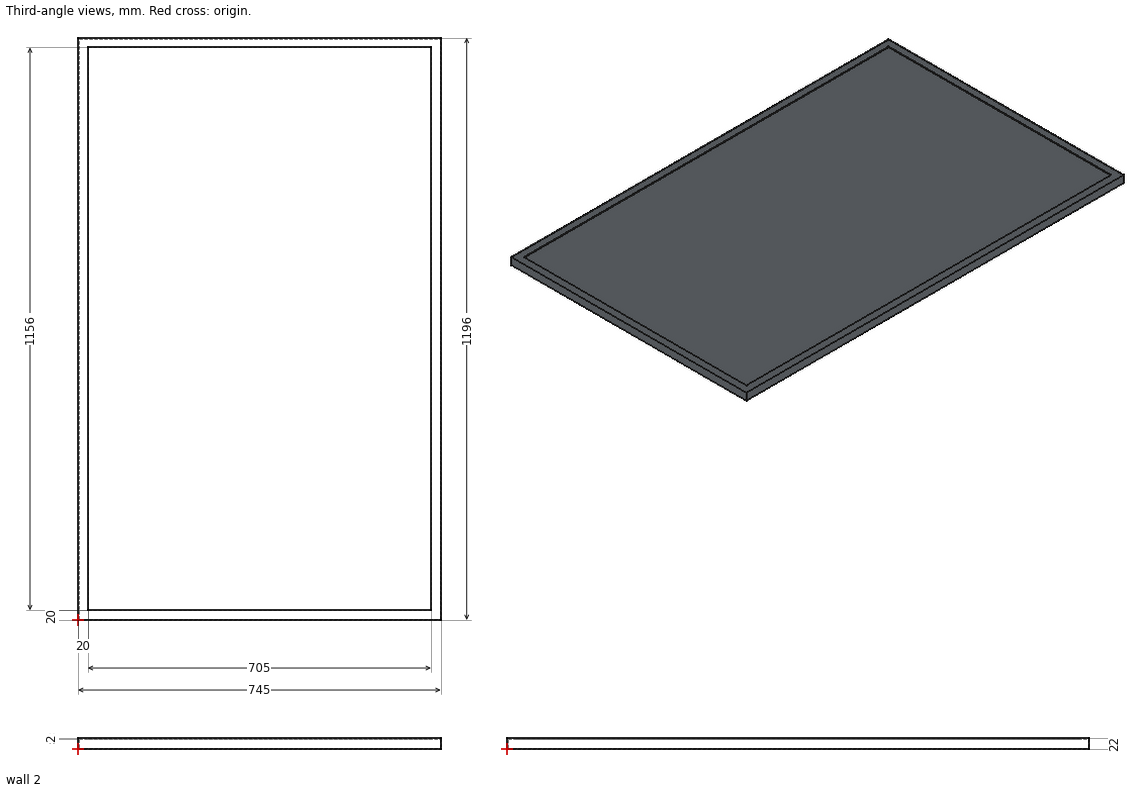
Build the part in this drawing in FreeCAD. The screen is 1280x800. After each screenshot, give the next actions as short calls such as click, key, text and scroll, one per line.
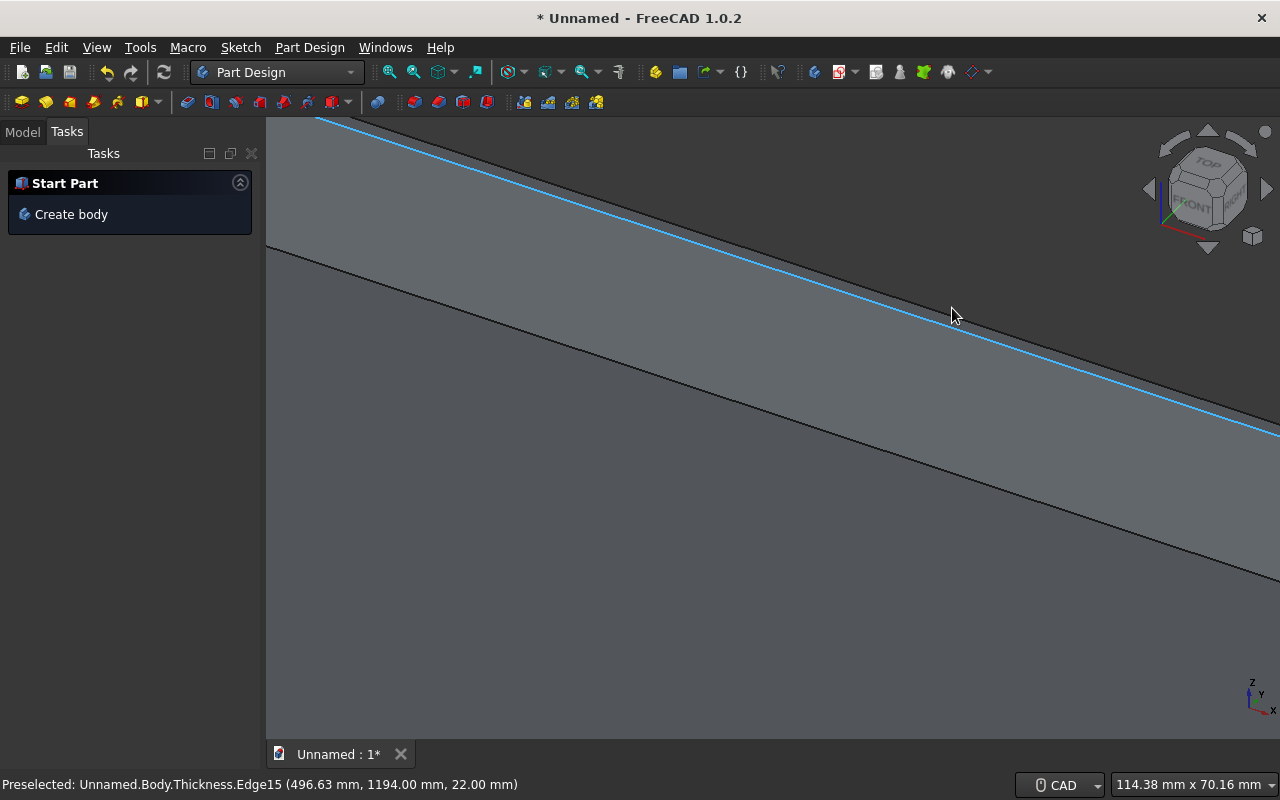
scroll(942, 320, up, 4)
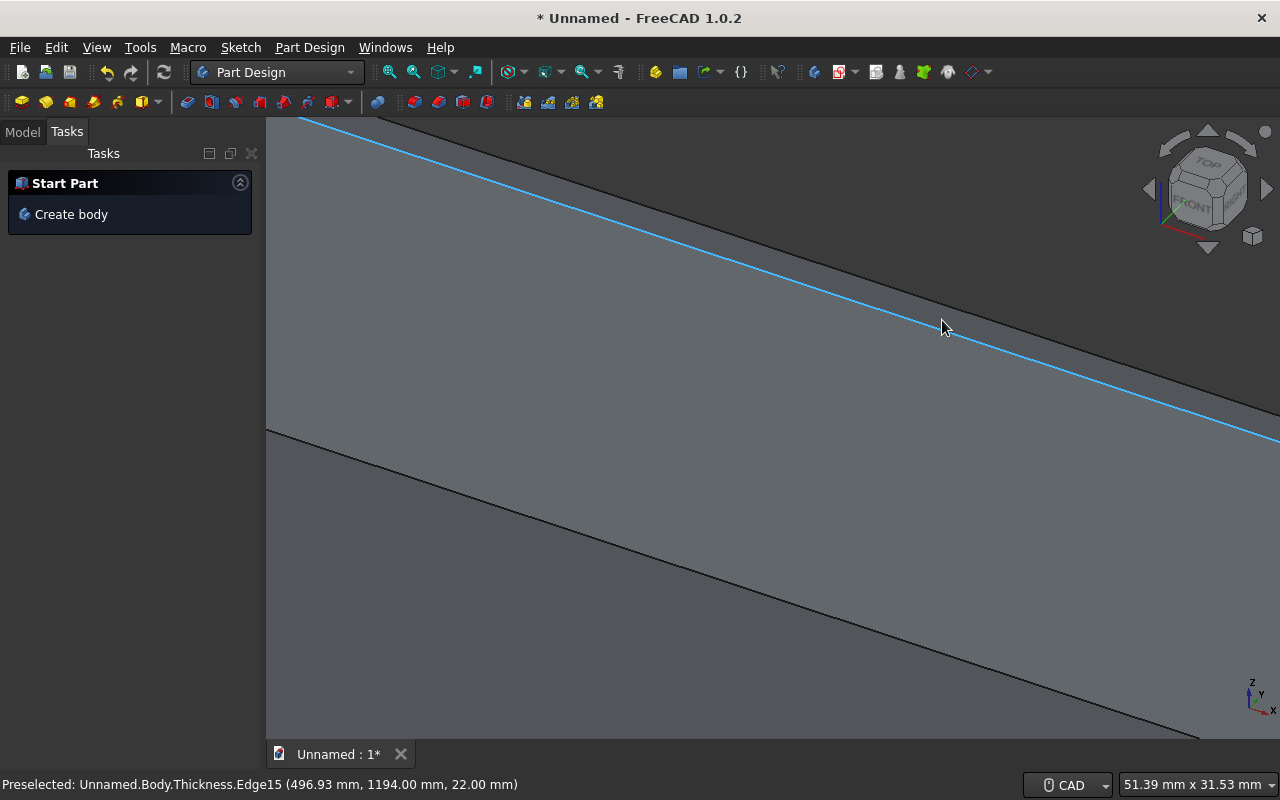
click(390, 72)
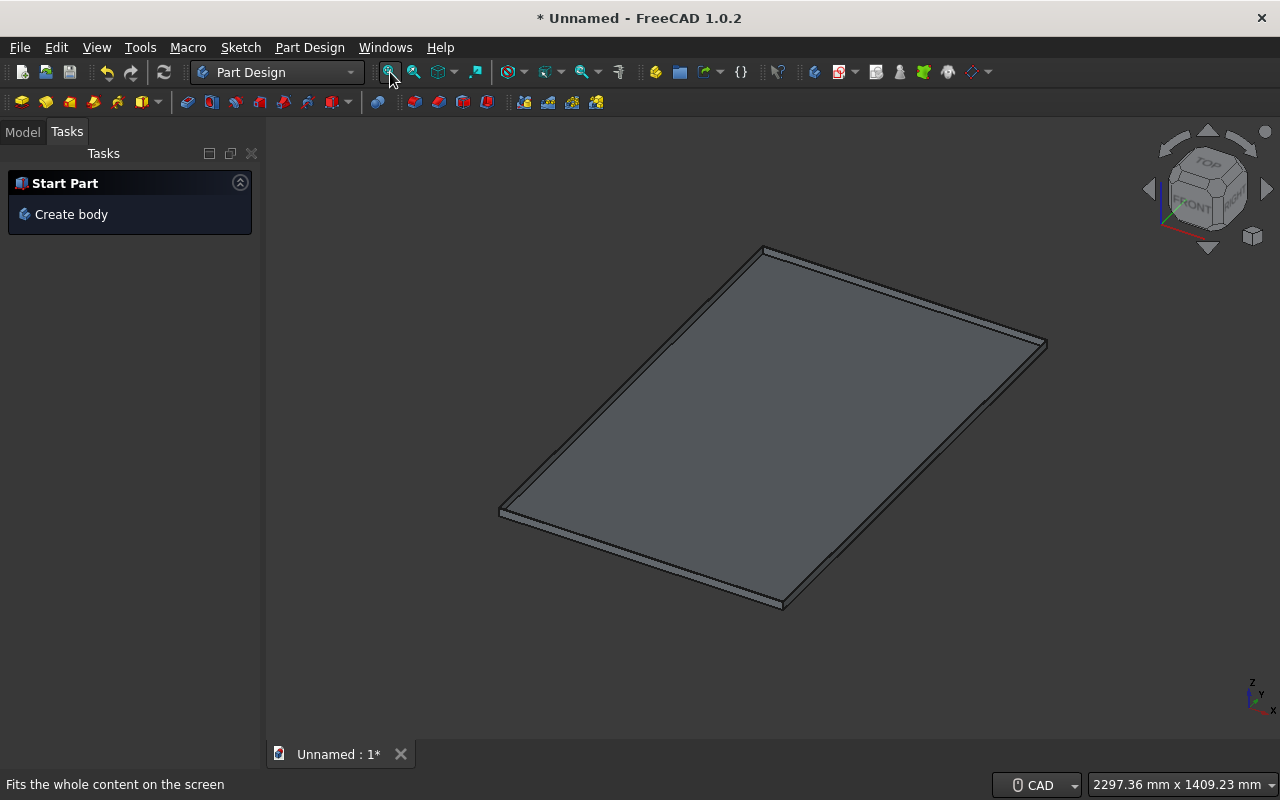
key(0)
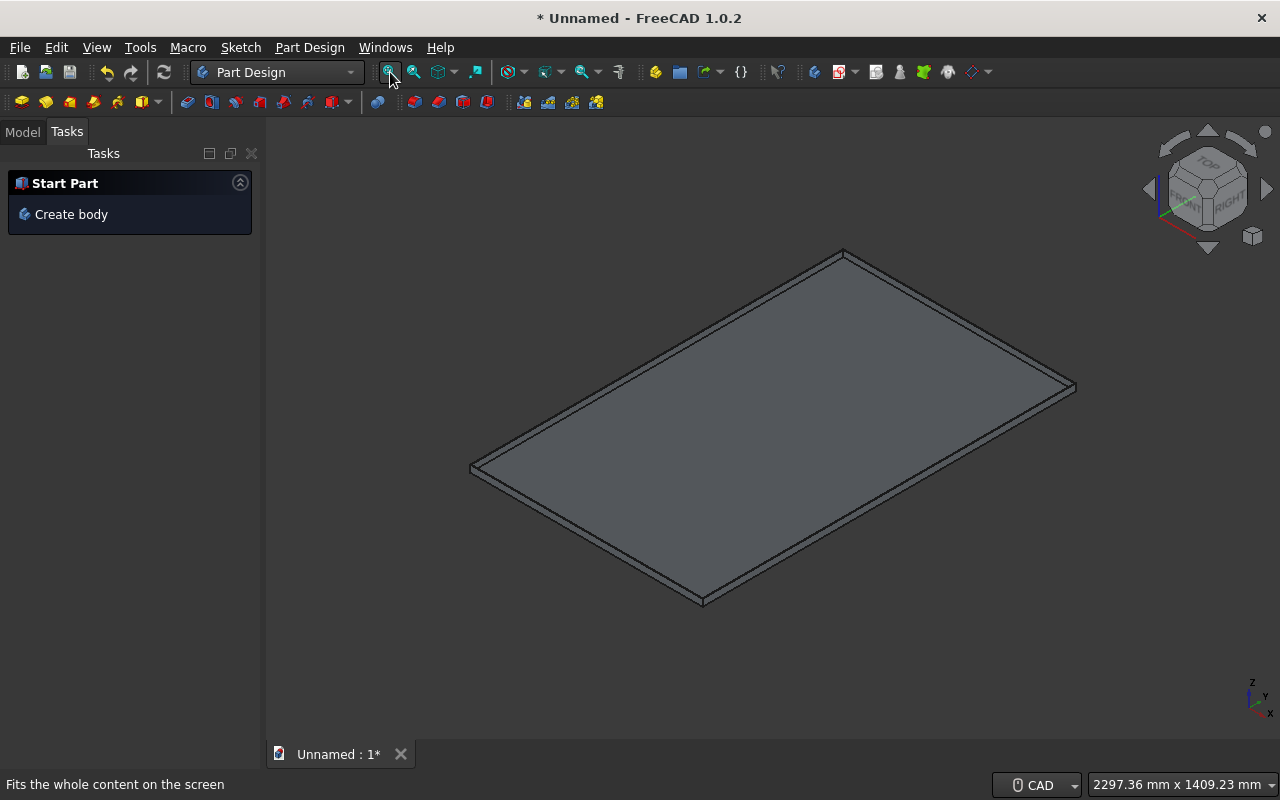
scroll(998, 338, up, 15)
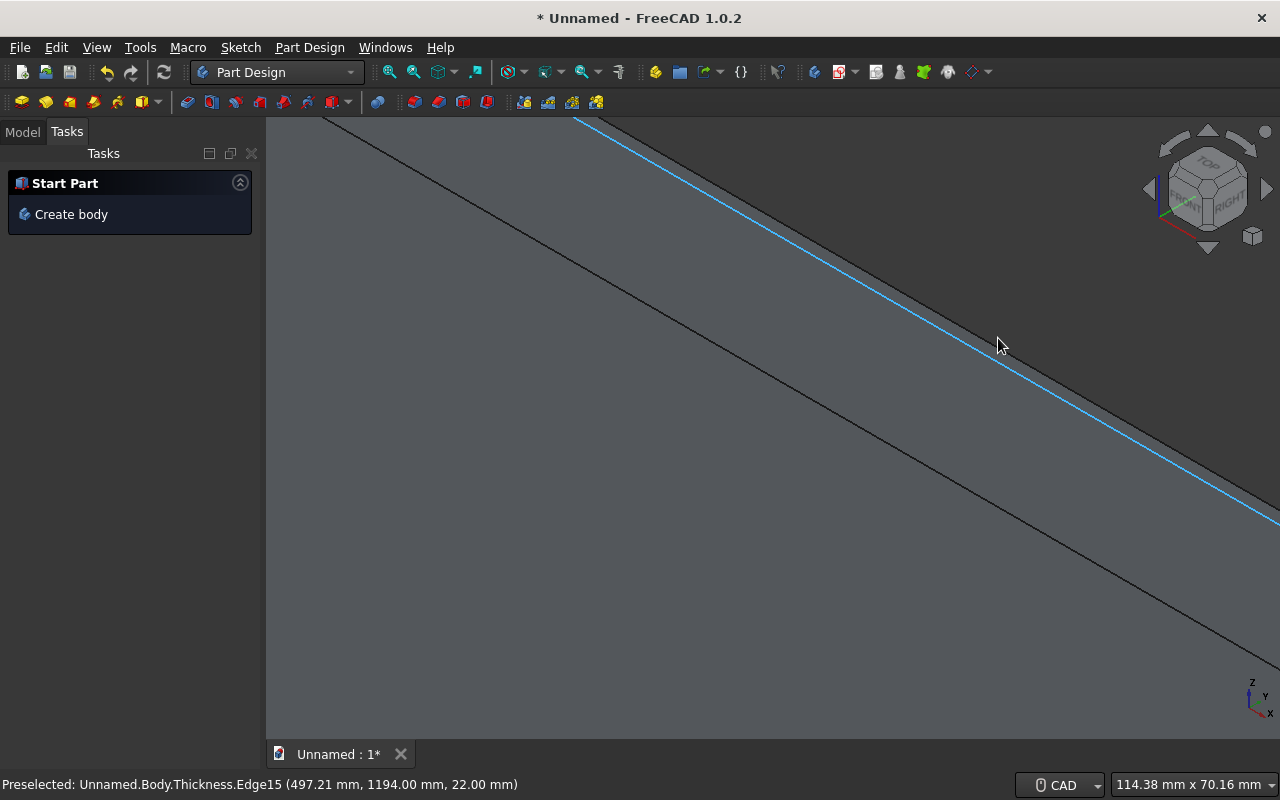
scroll(984, 348, up, 4)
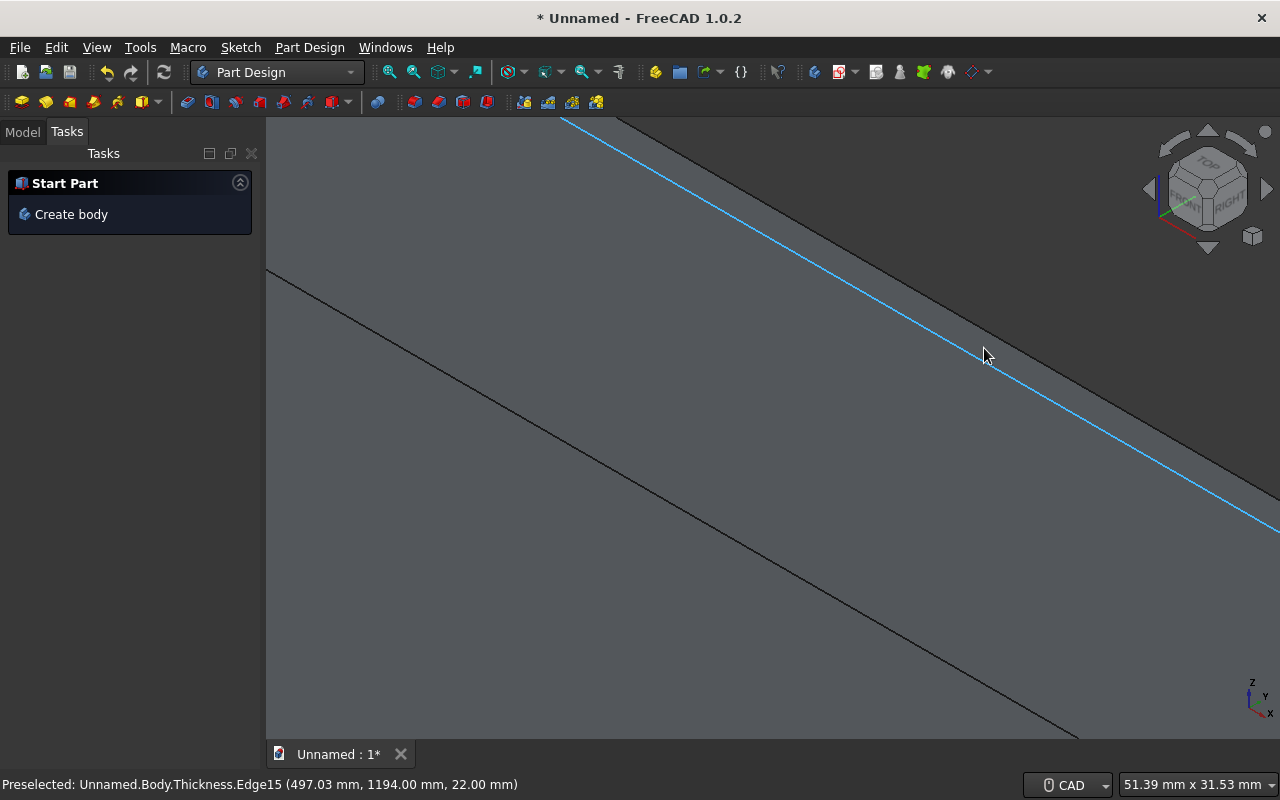
click(982, 349)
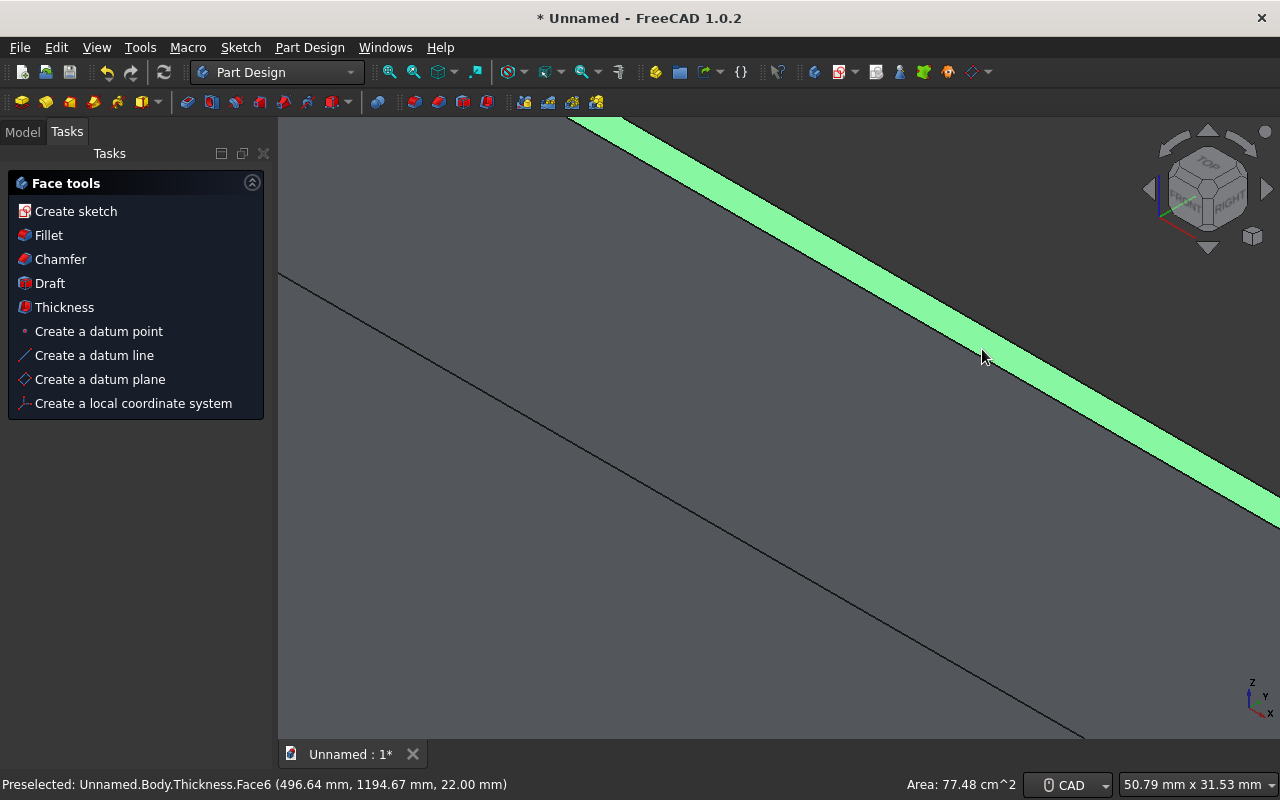
click(840, 72)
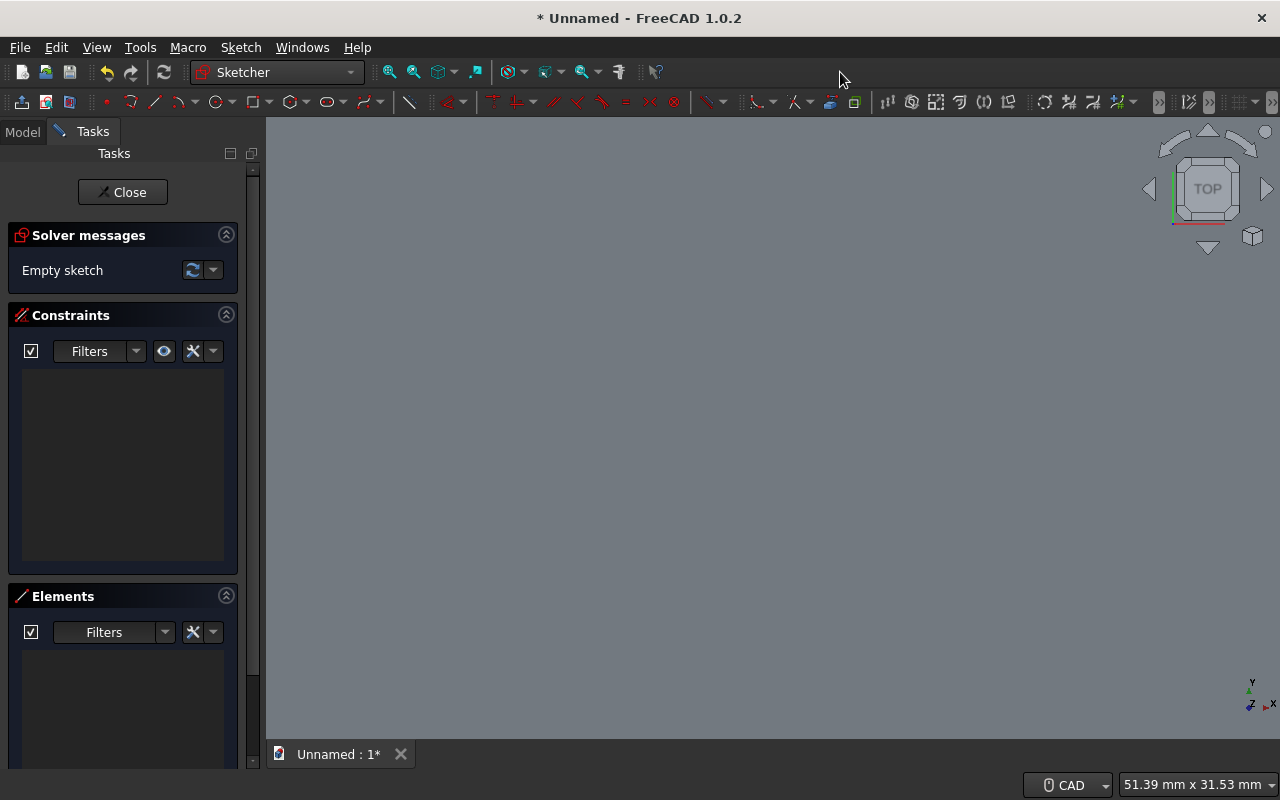
scroll(704, 428, down, 15)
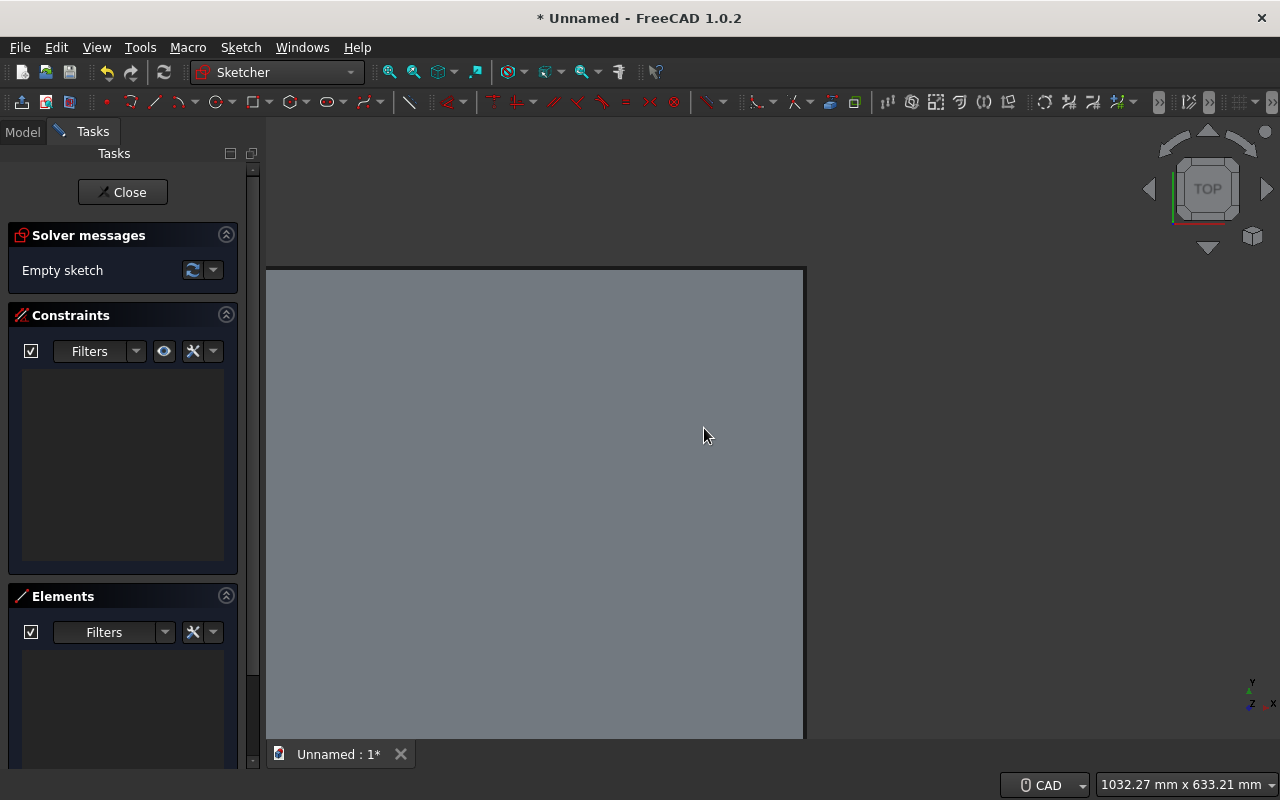
scroll(858, 180, down, 5)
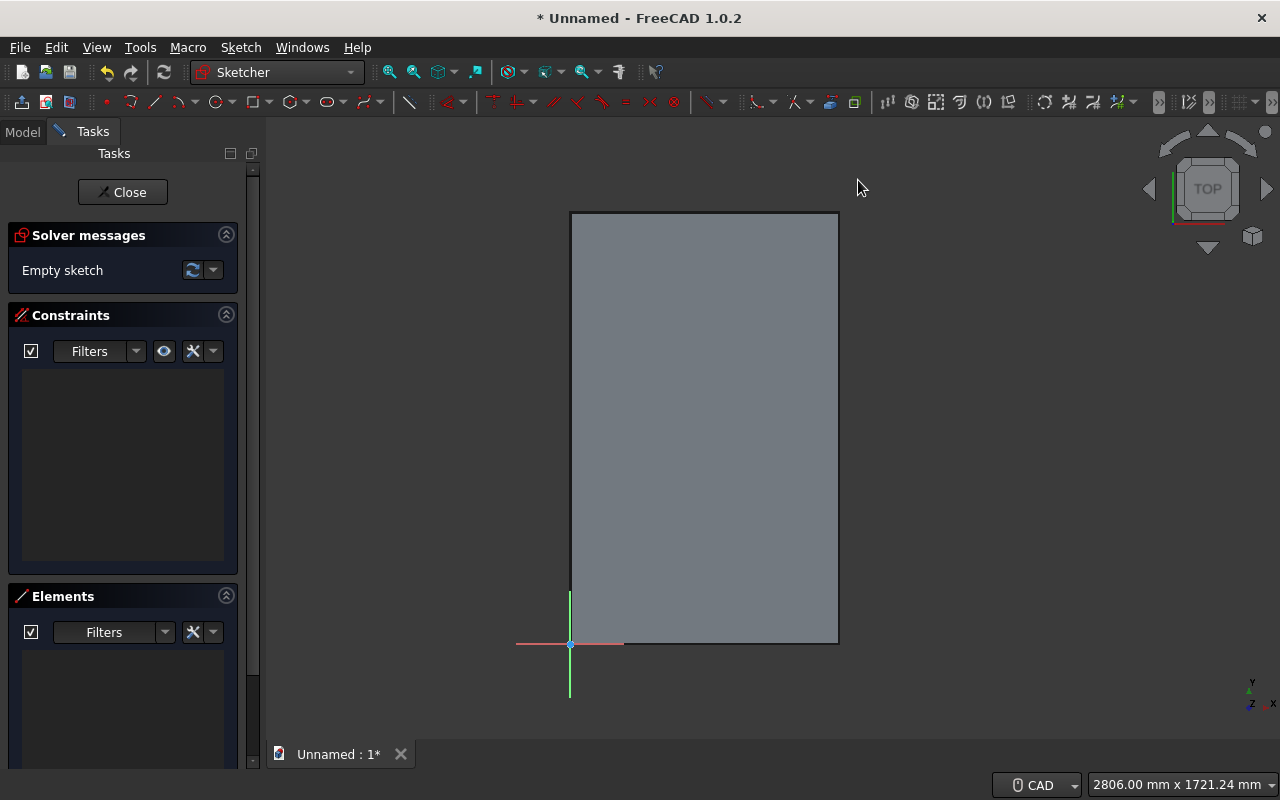
click(254, 102)